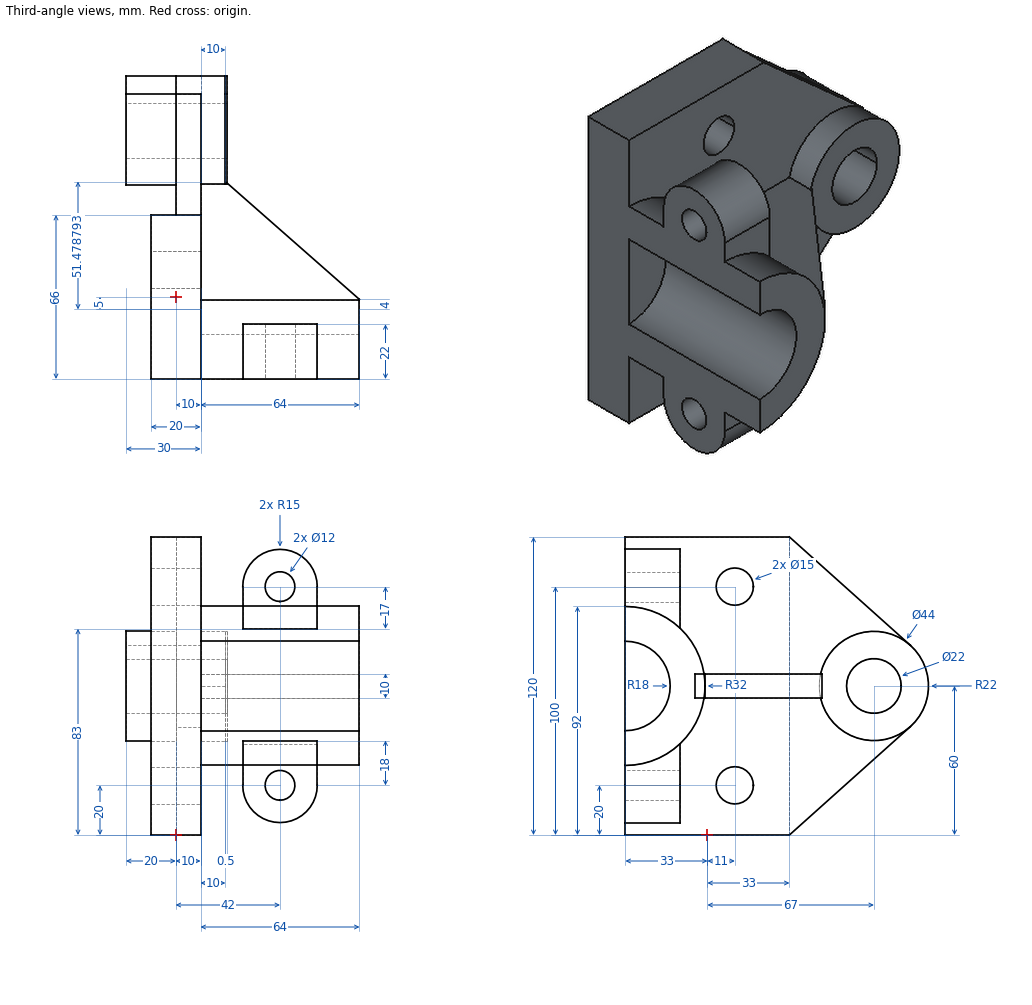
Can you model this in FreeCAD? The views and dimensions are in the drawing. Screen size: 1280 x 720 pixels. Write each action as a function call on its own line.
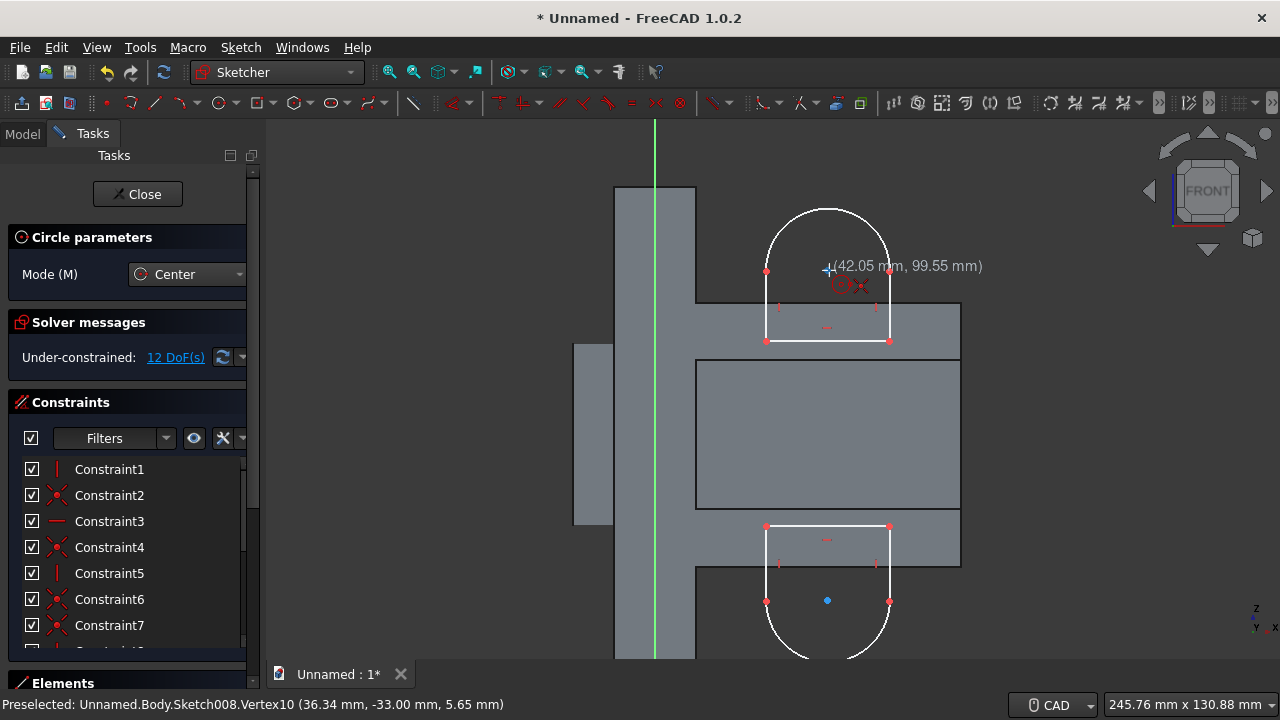
click(829, 269)
click(846, 252)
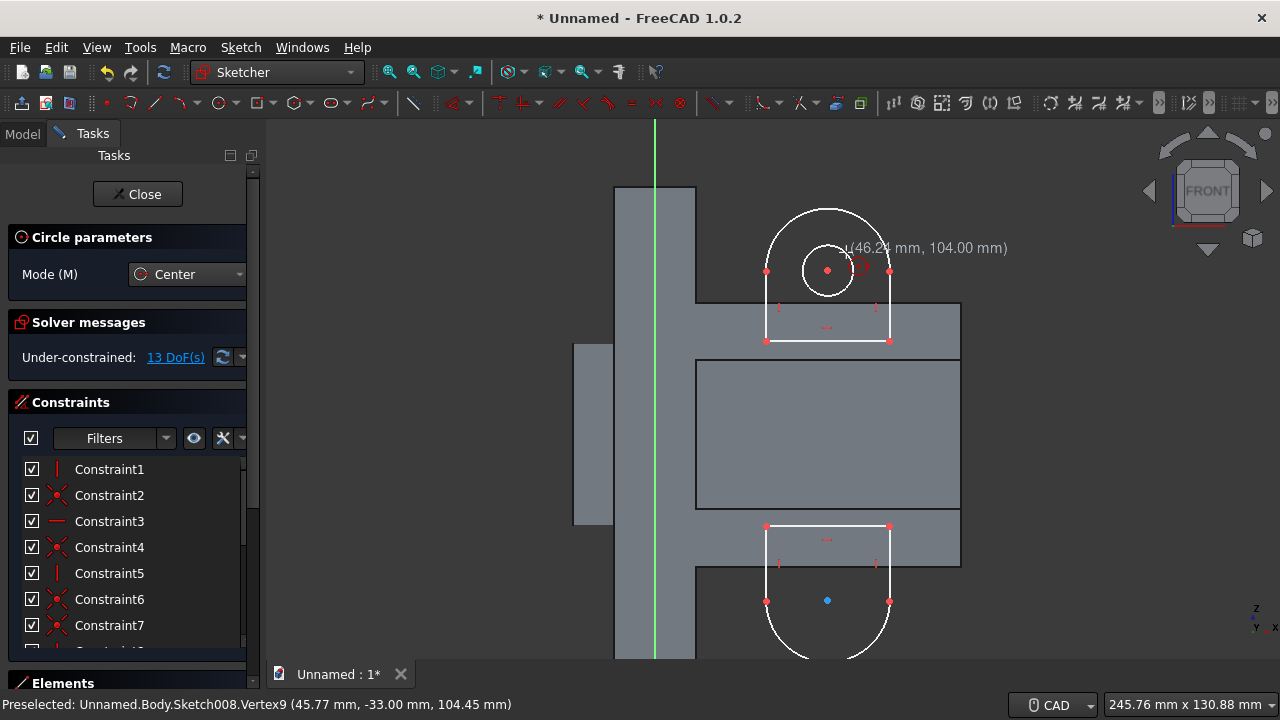
click(829, 600)
click(846, 582)
key(Escape)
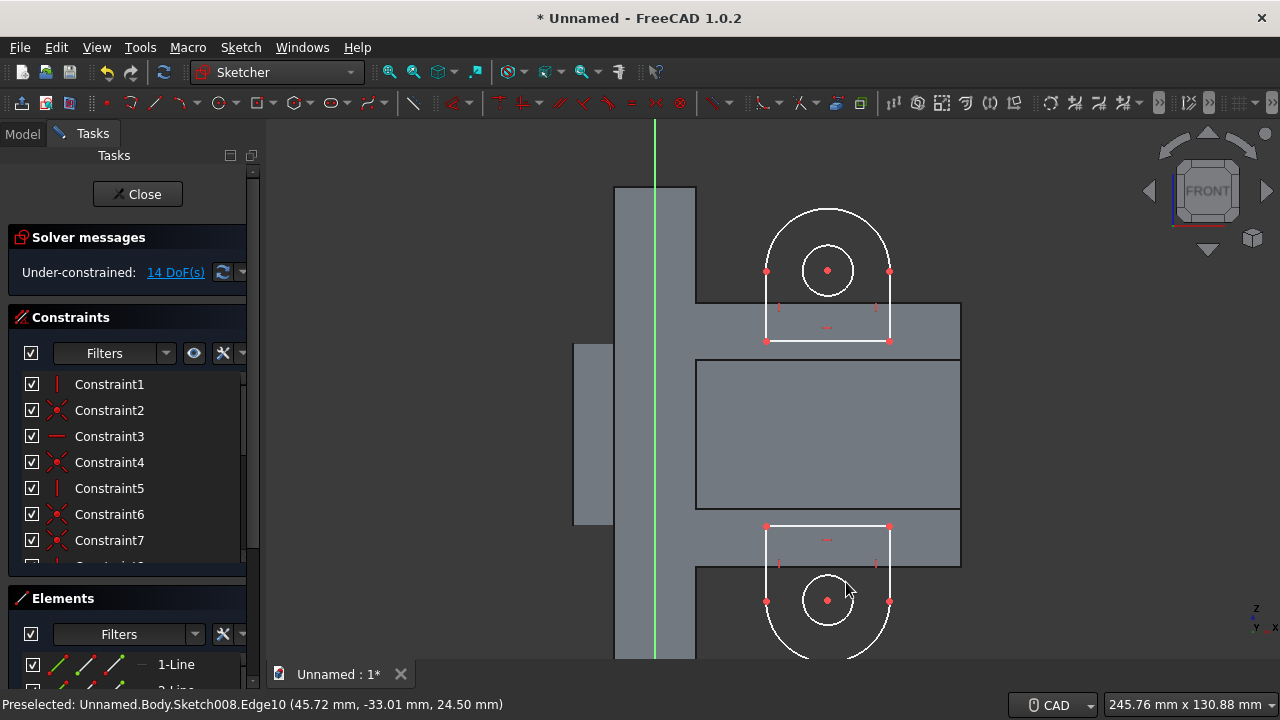
click(766, 292)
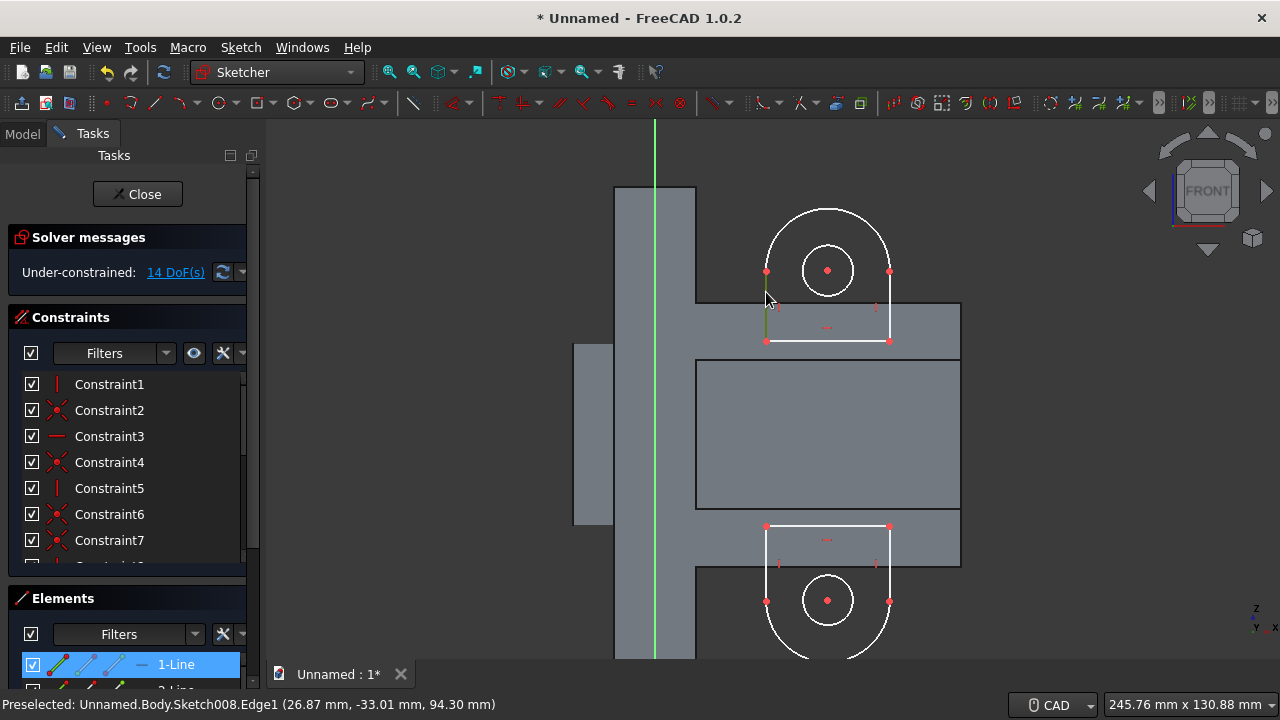
click(865, 221)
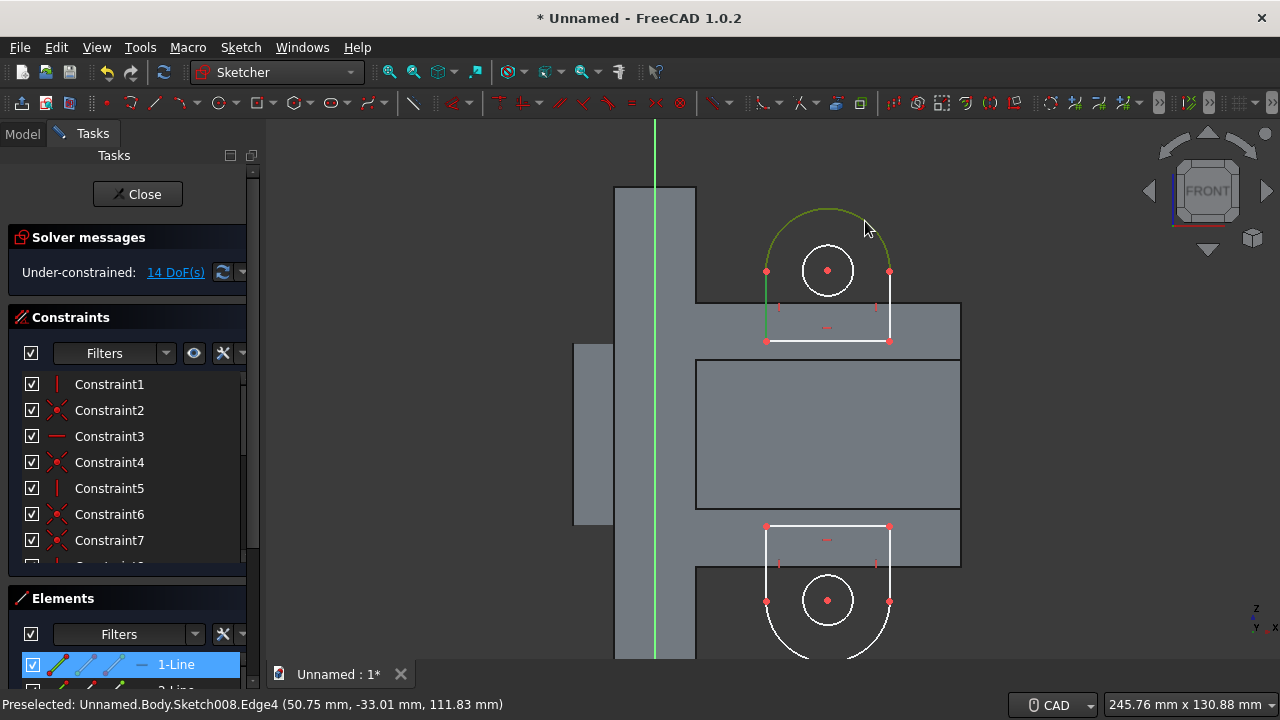
click(608, 104)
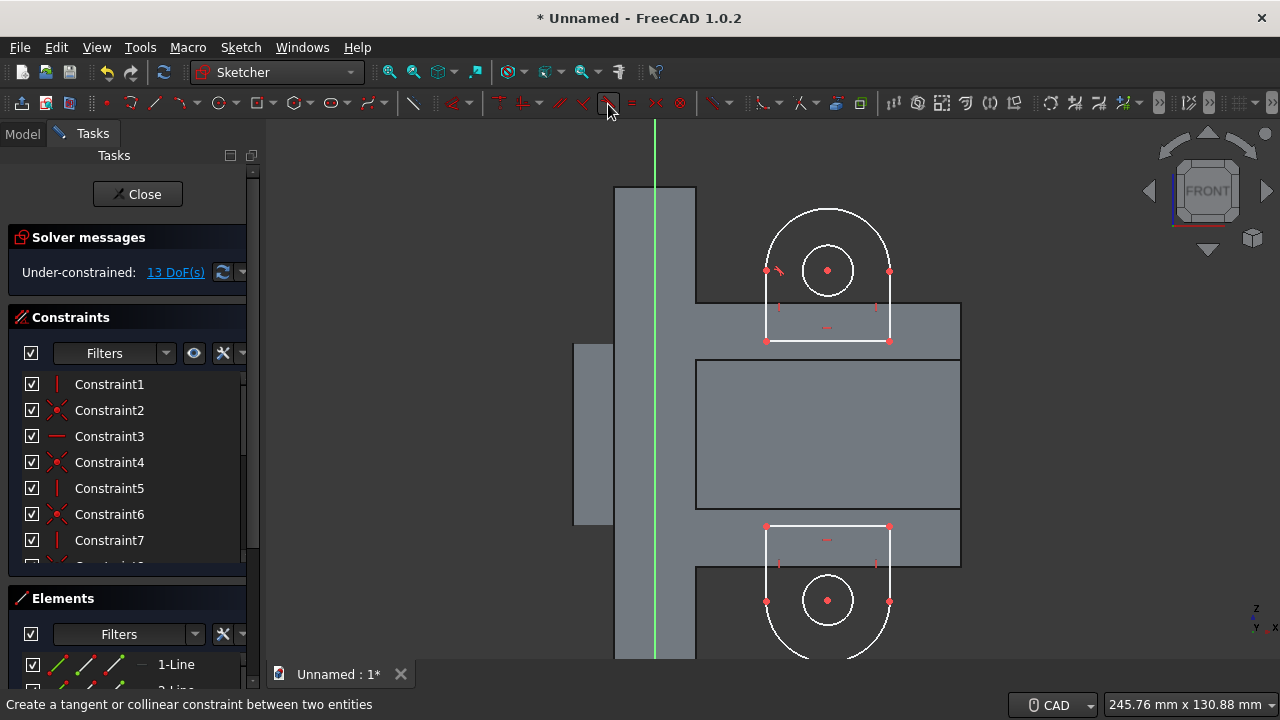
click(890, 320)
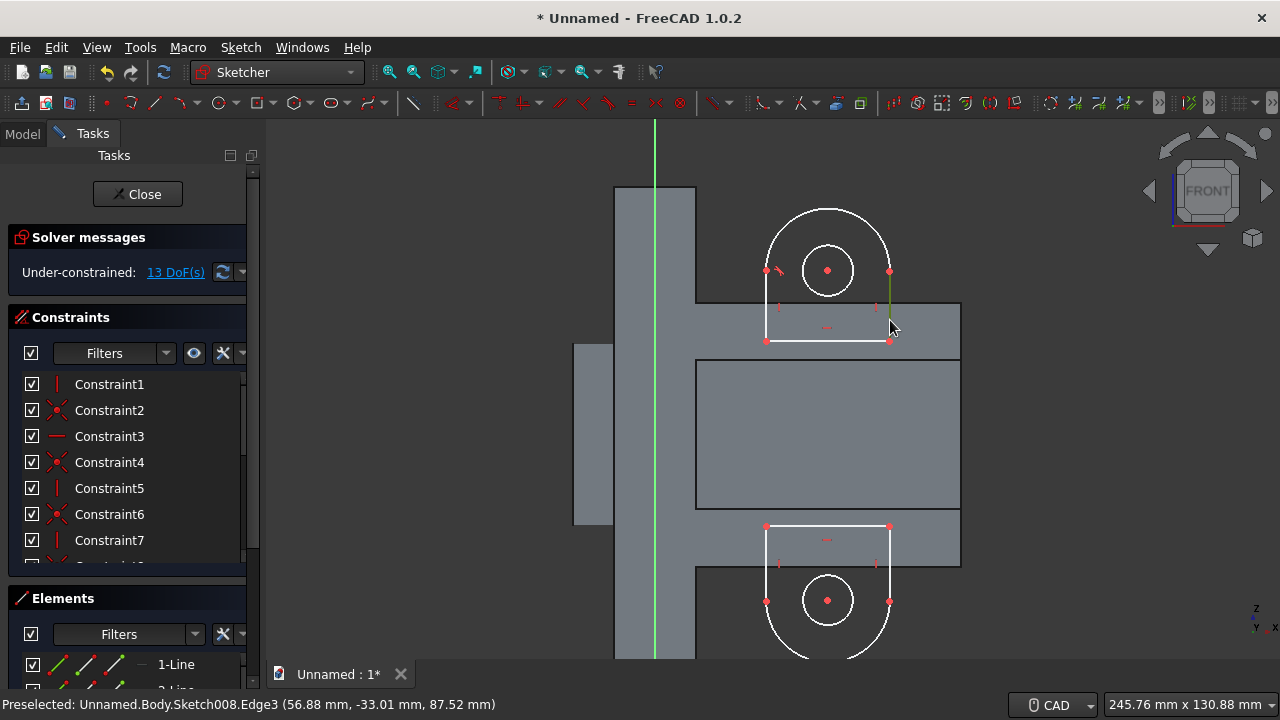
click(865, 221)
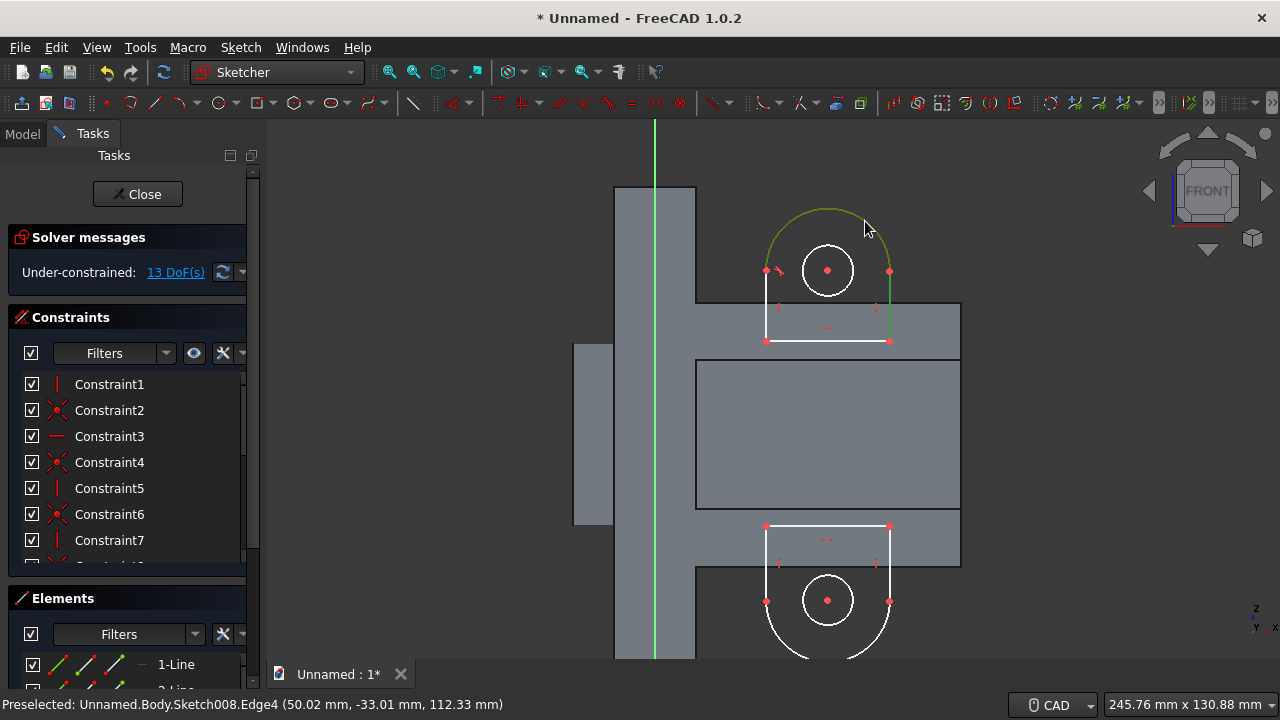
click(608, 104)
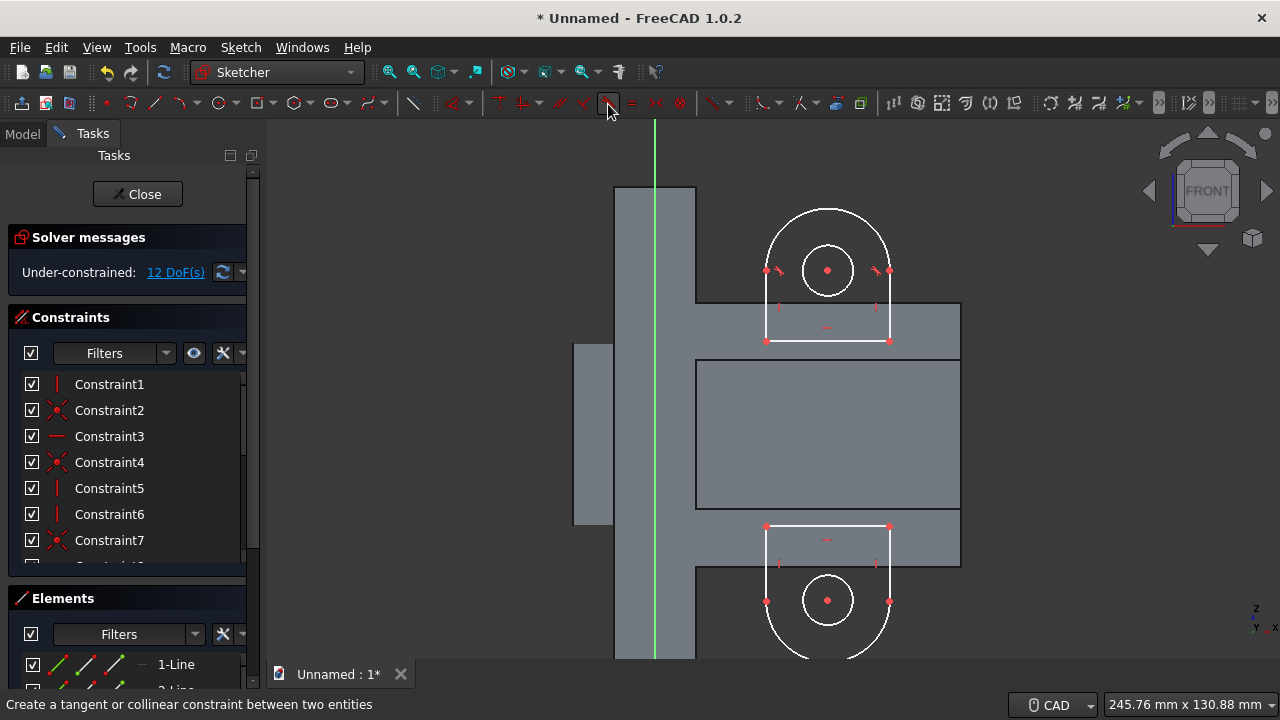
click(890, 579)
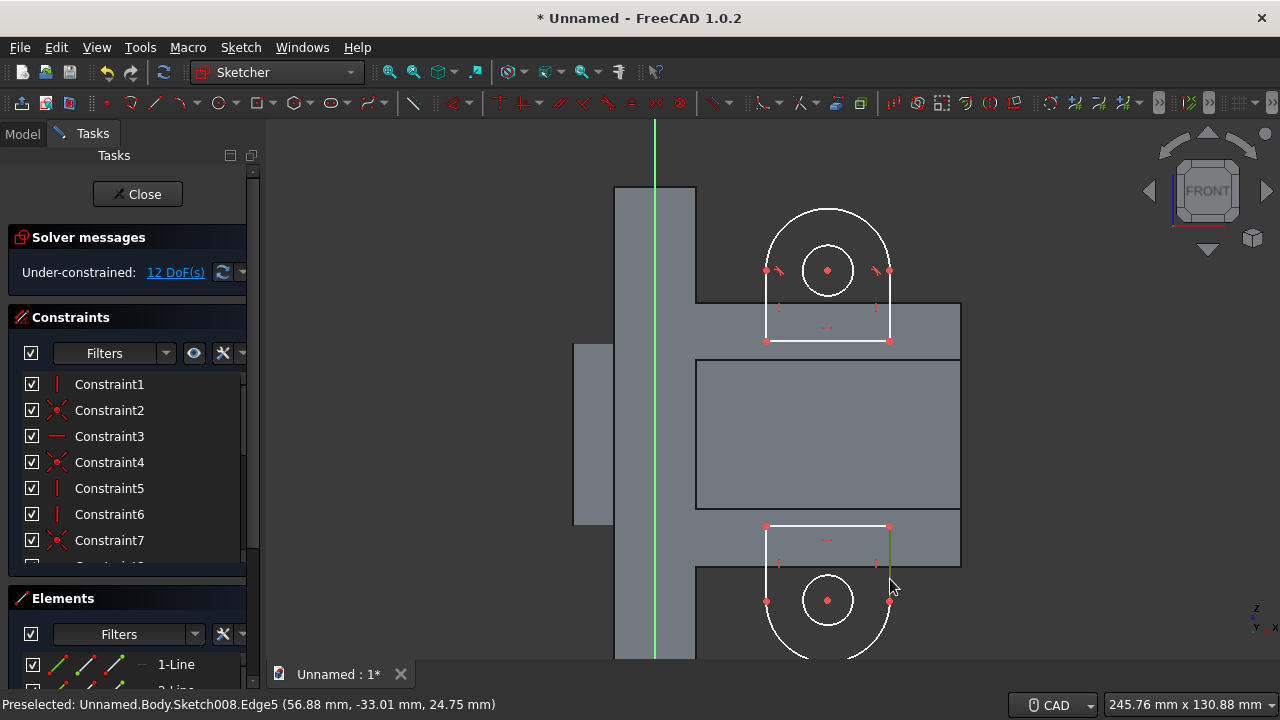
scroll(566, 275, down, 2)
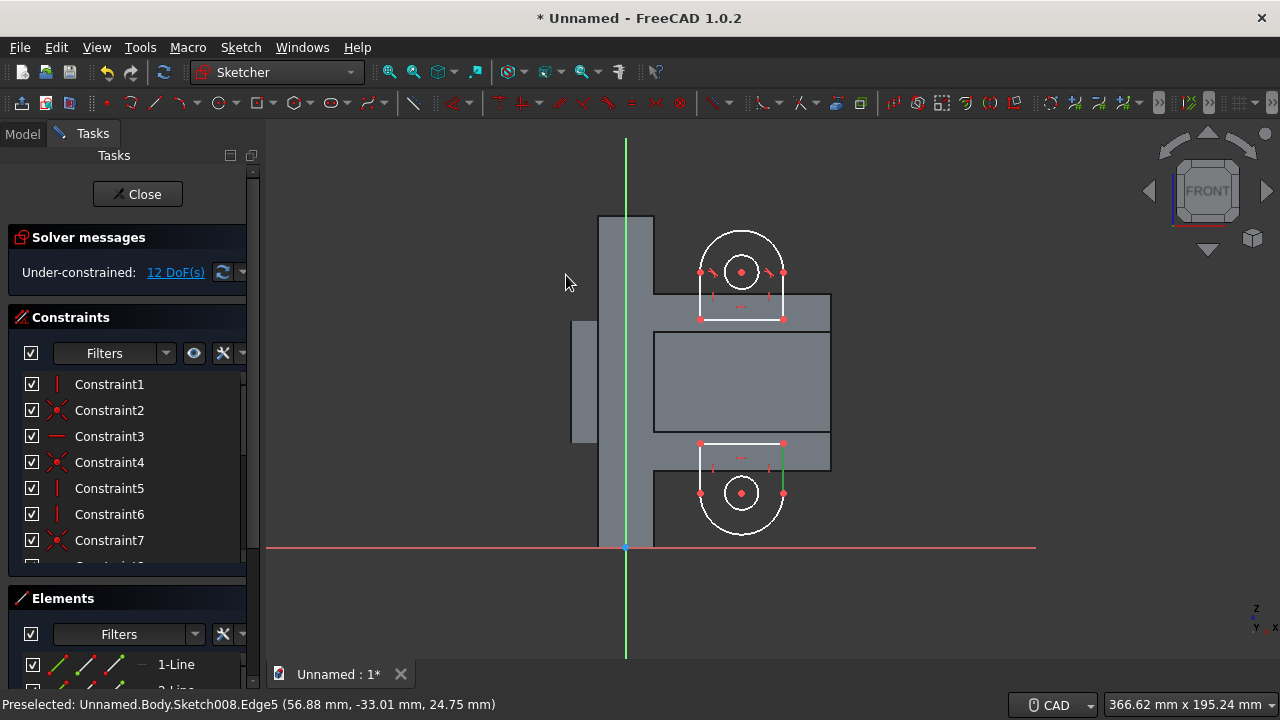
click(718, 527)